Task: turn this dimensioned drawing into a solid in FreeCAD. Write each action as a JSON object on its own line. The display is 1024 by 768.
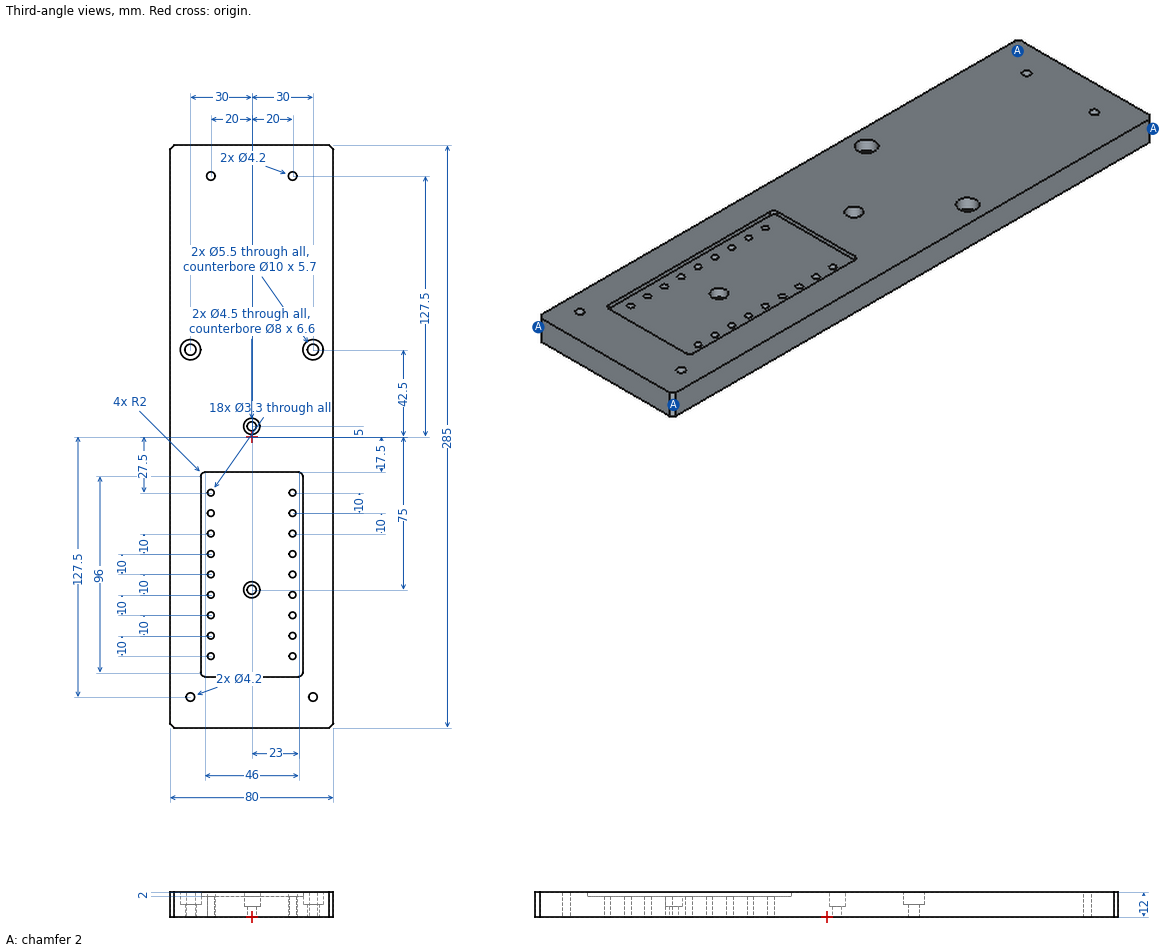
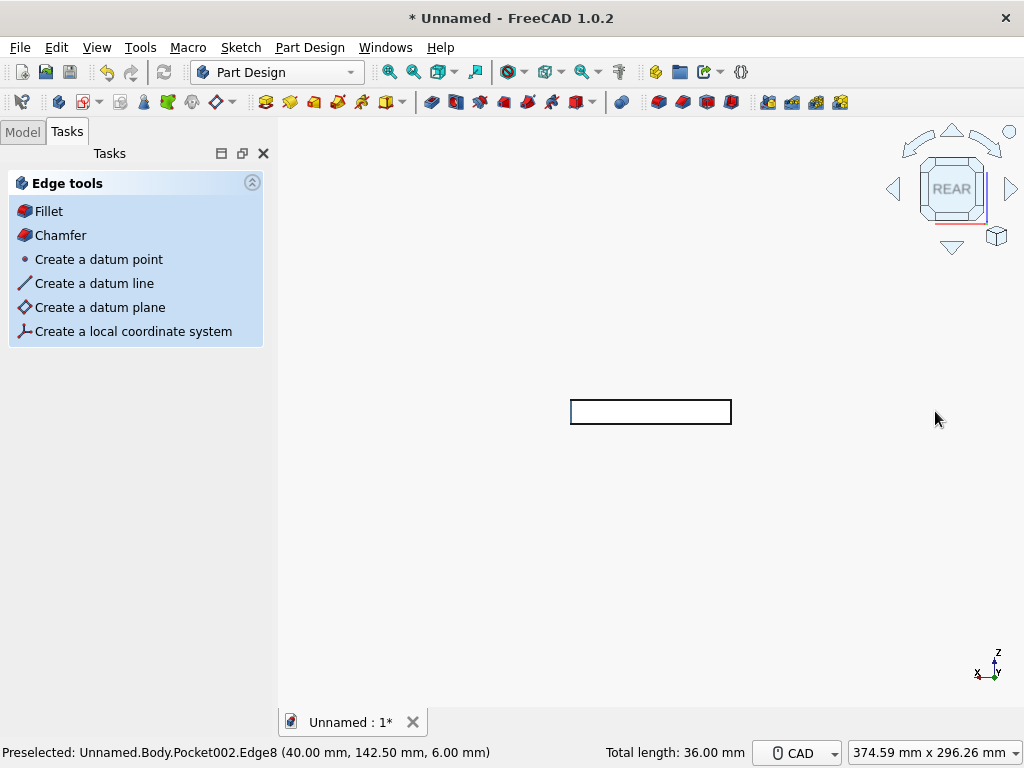
{"action": "left_click", "coordinate": [731, 411], "text": "ctrl"}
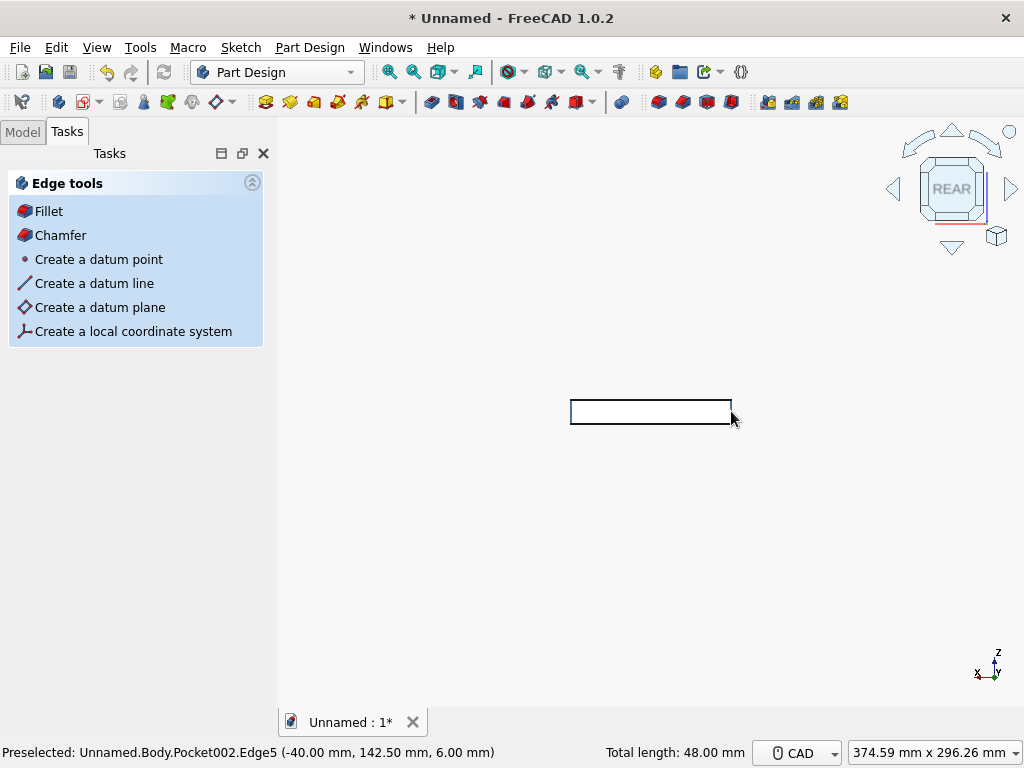
{"action": "left_click", "coordinate": [684, 102]}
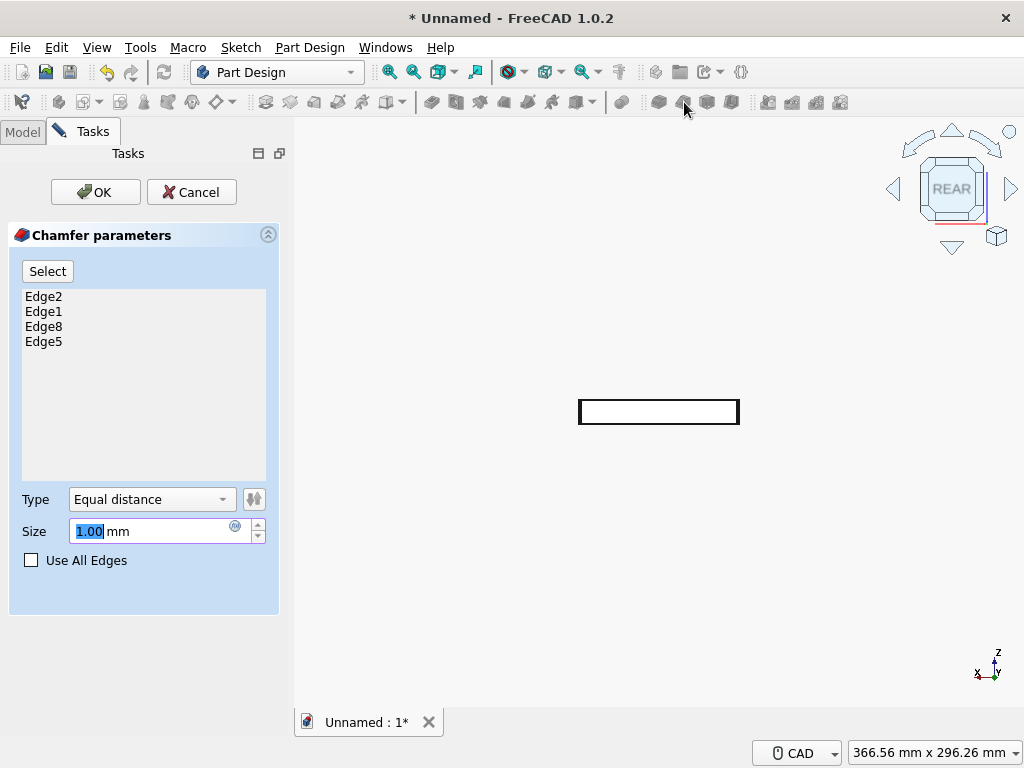
{"action": "type", "text": "2"}
{"action": "key", "text": "Tab"}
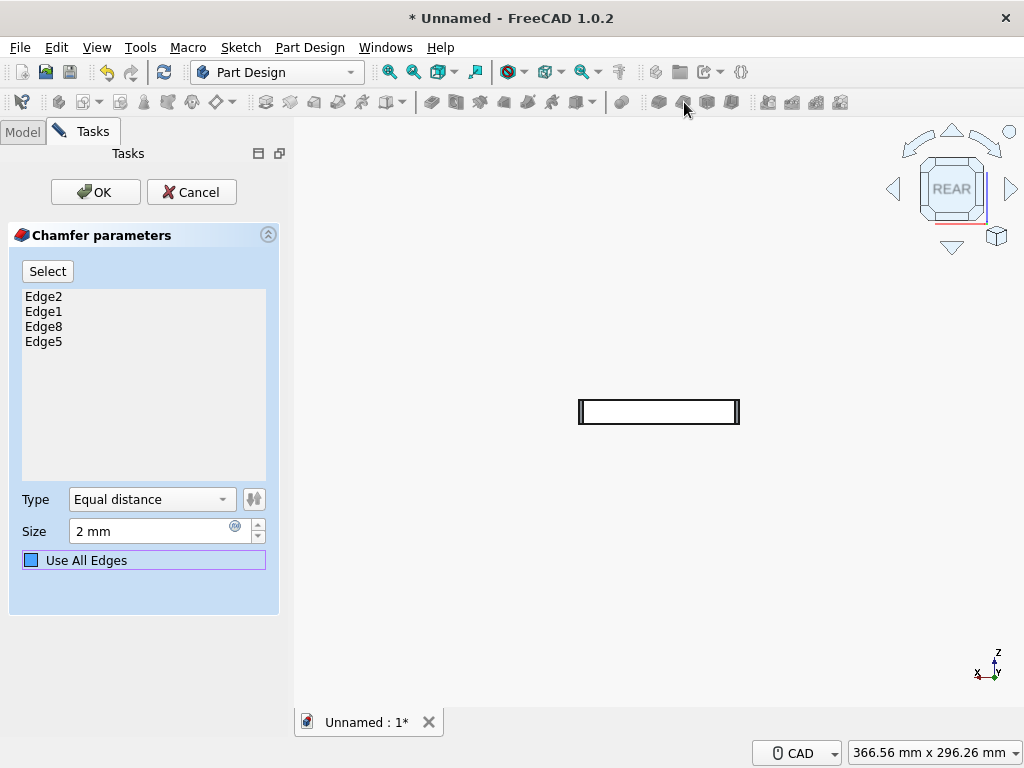
{"action": "left_click", "coordinate": [96, 192]}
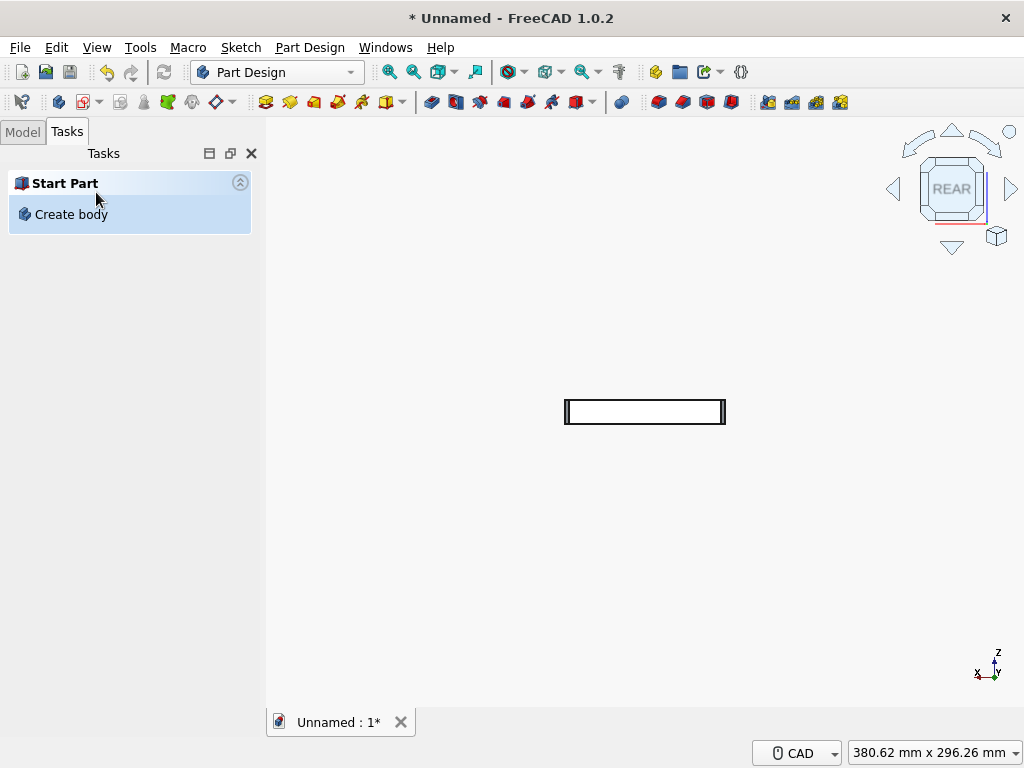
{"action": "key", "text": "v f"}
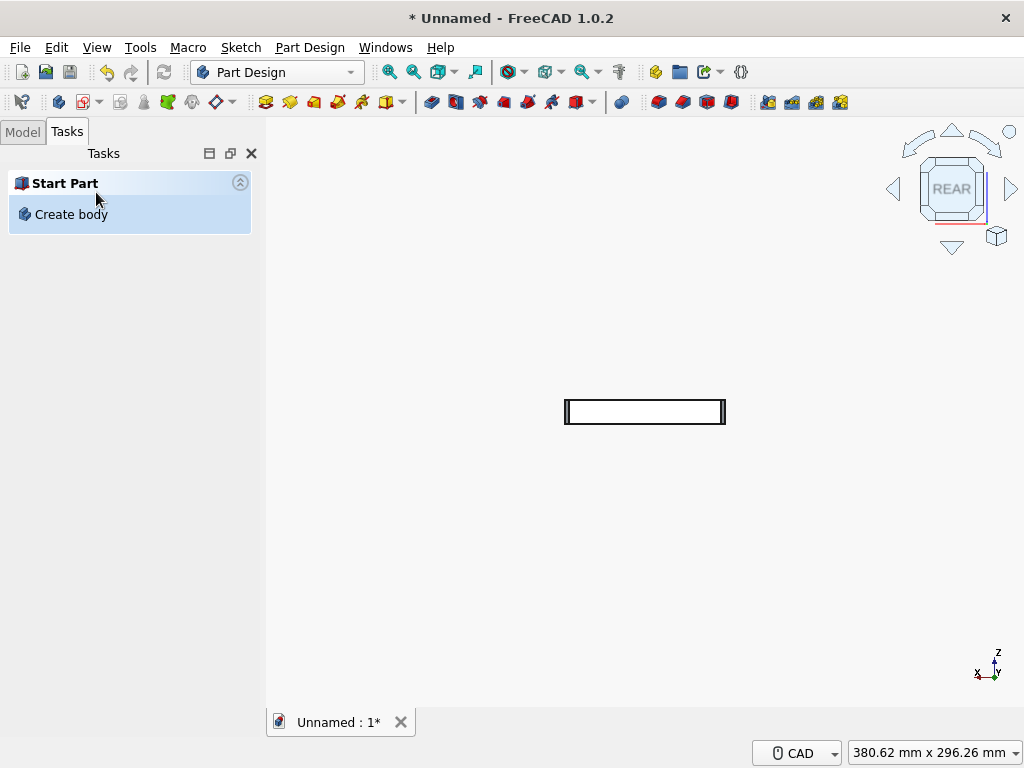
{"action": "key", "text": "0"}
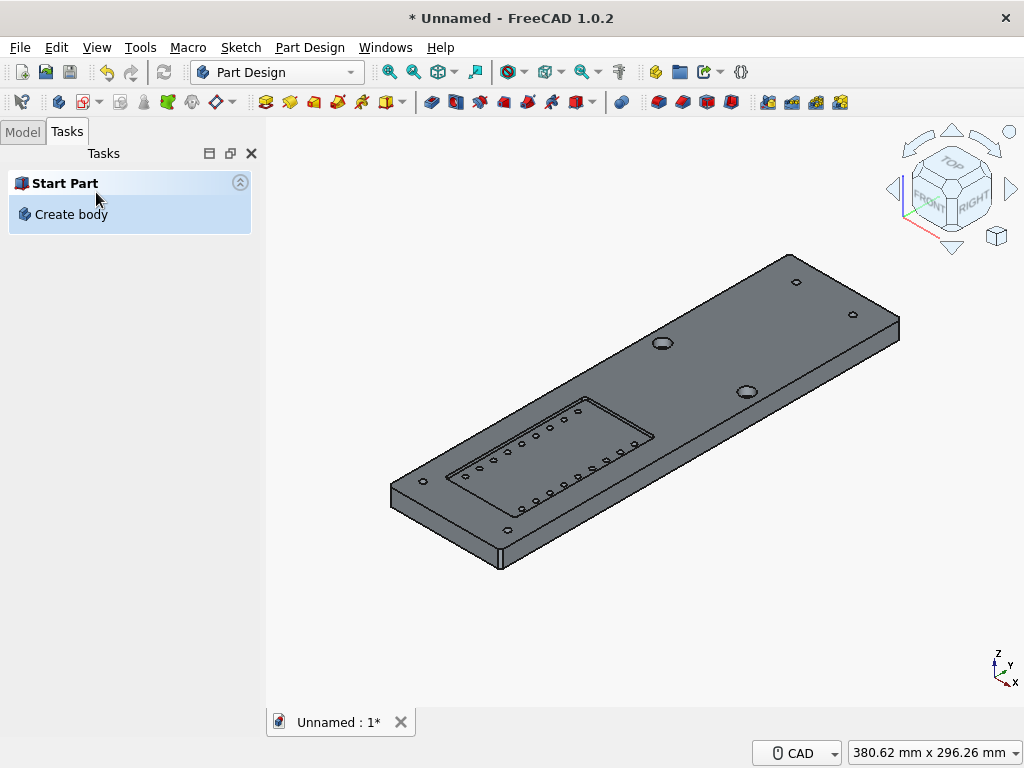
{"action": "left_click", "coordinate": [760, 335]}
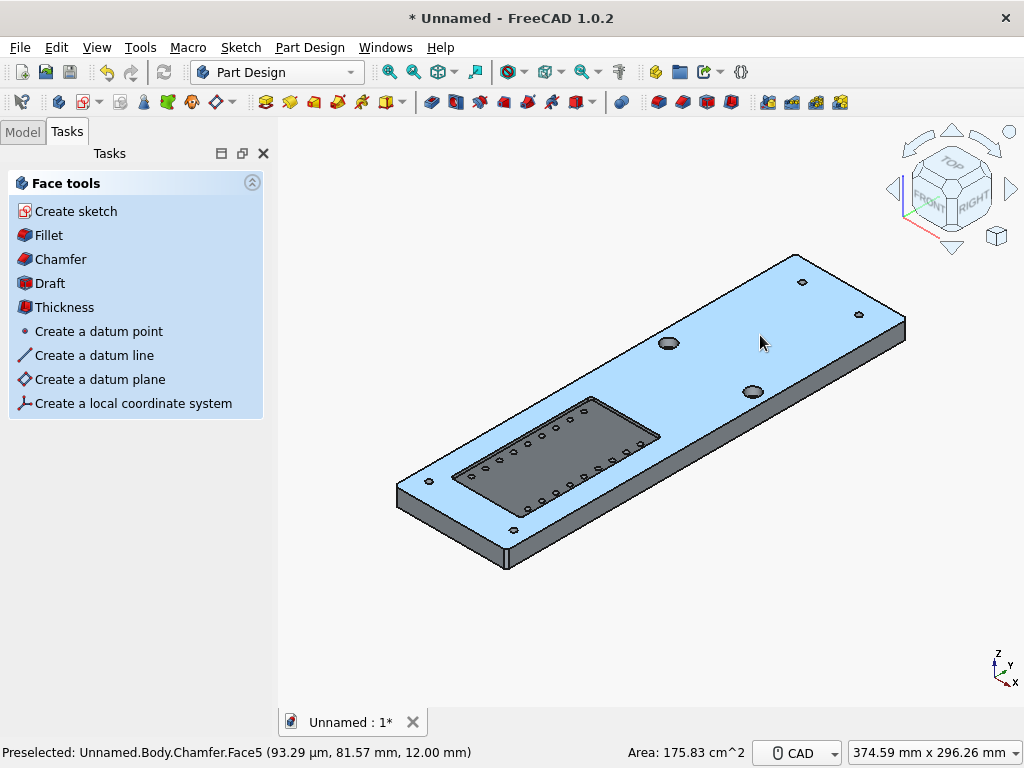
{"action": "left_click", "coordinate": [84, 102]}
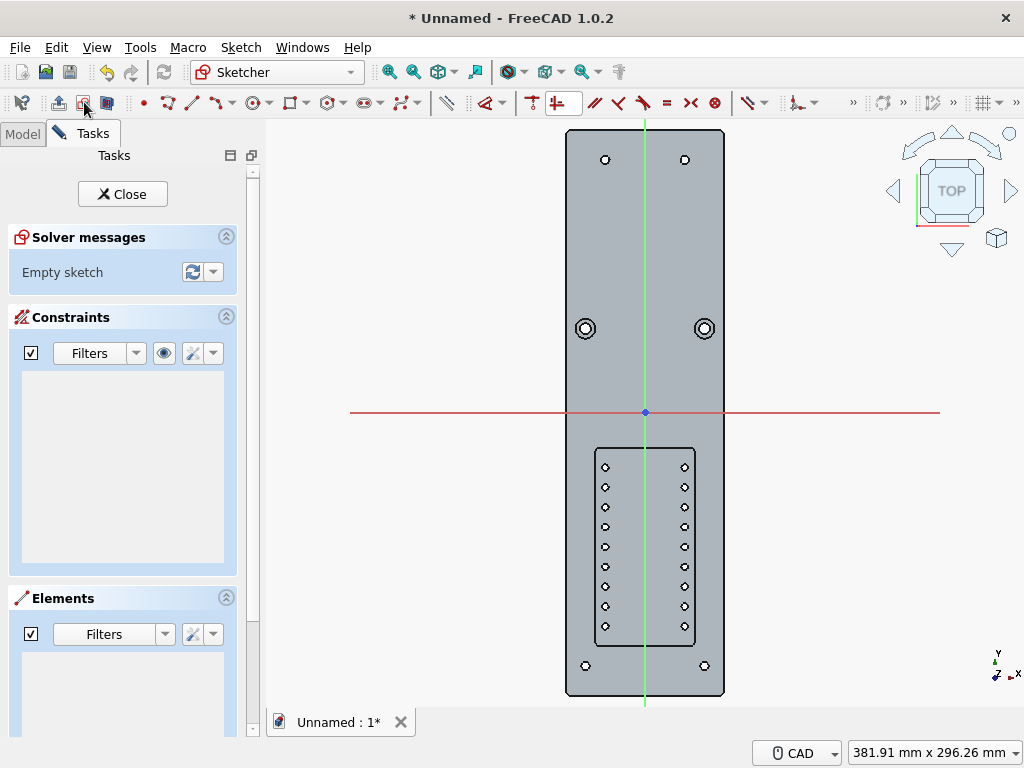
{"action": "scroll", "coordinate": [701, 539], "scroll_direction": "up", "scroll_amount": 4}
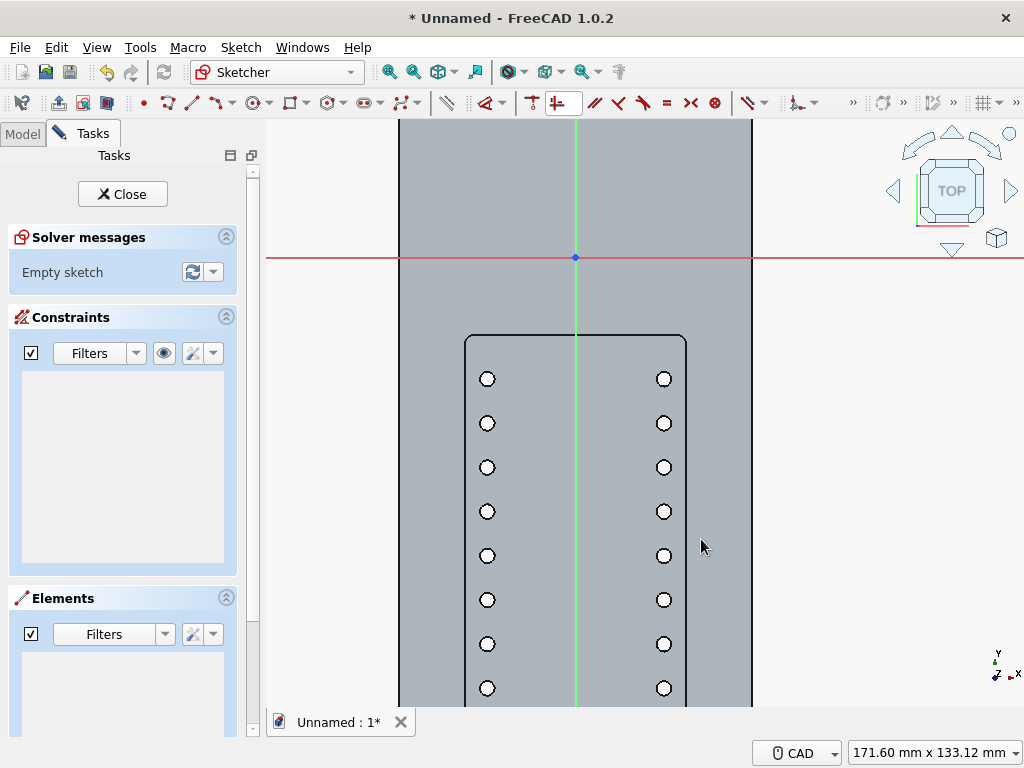
{"action": "key", "text": "g c"}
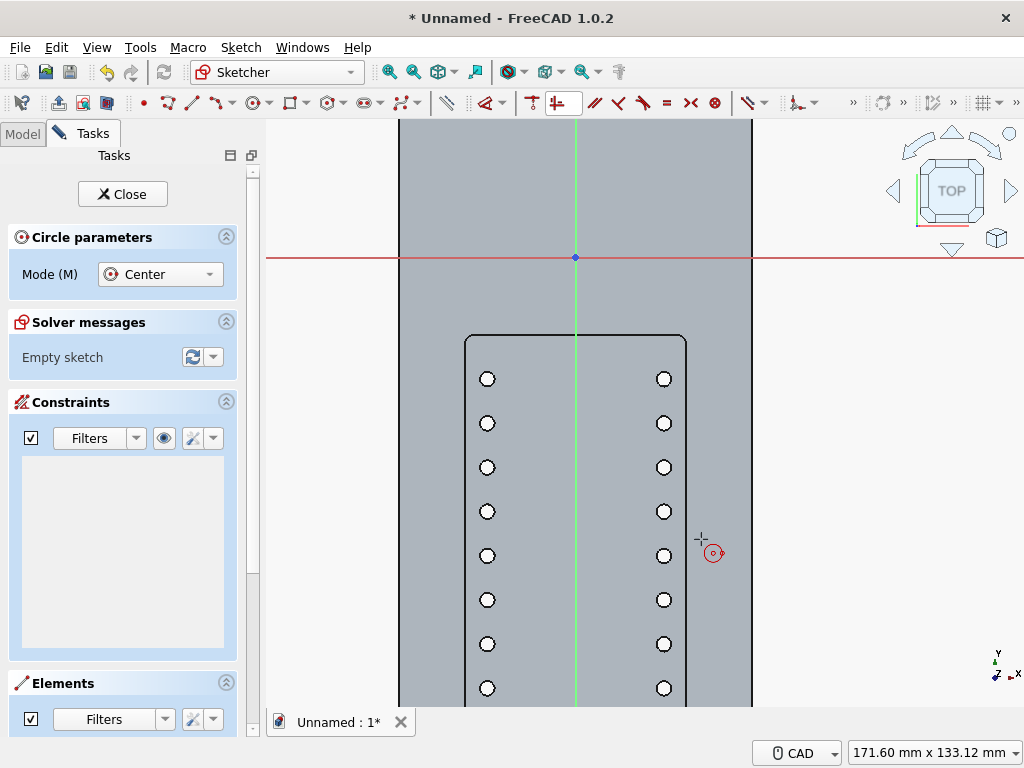
{"action": "scroll", "coordinate": [576, 236], "scroll_direction": "up", "scroll_amount": 5}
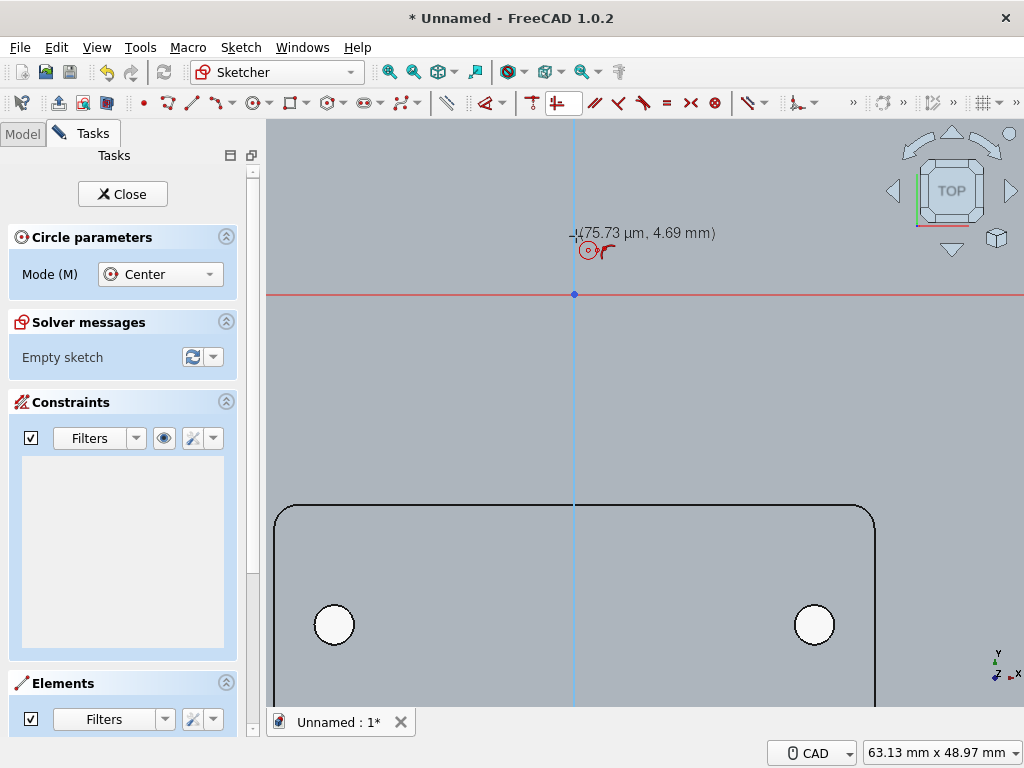
{"action": "left_click", "coordinate": [574, 235]}
{"action": "left_click", "coordinate": [593, 216]}